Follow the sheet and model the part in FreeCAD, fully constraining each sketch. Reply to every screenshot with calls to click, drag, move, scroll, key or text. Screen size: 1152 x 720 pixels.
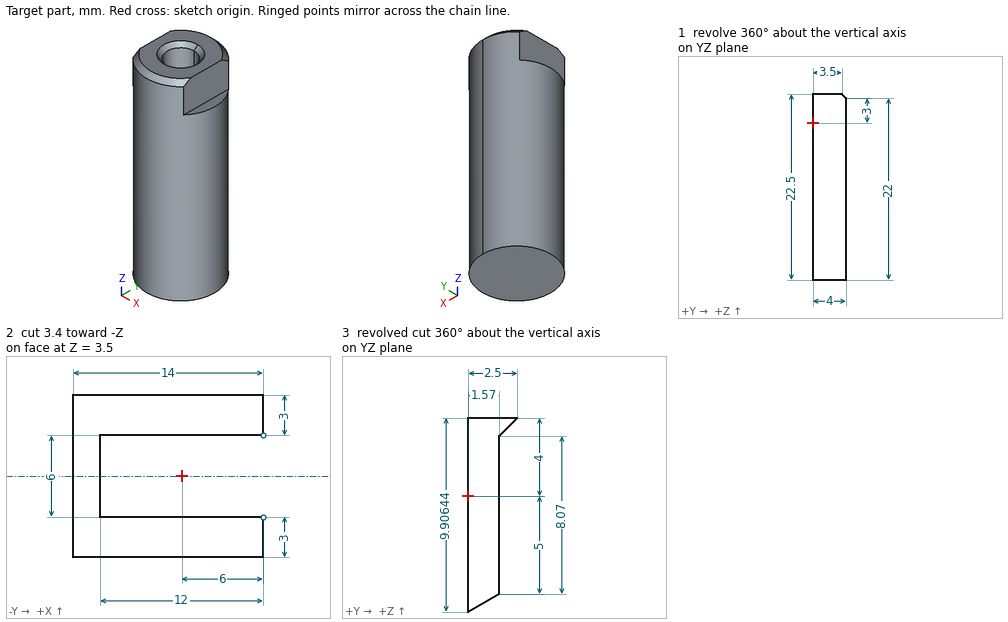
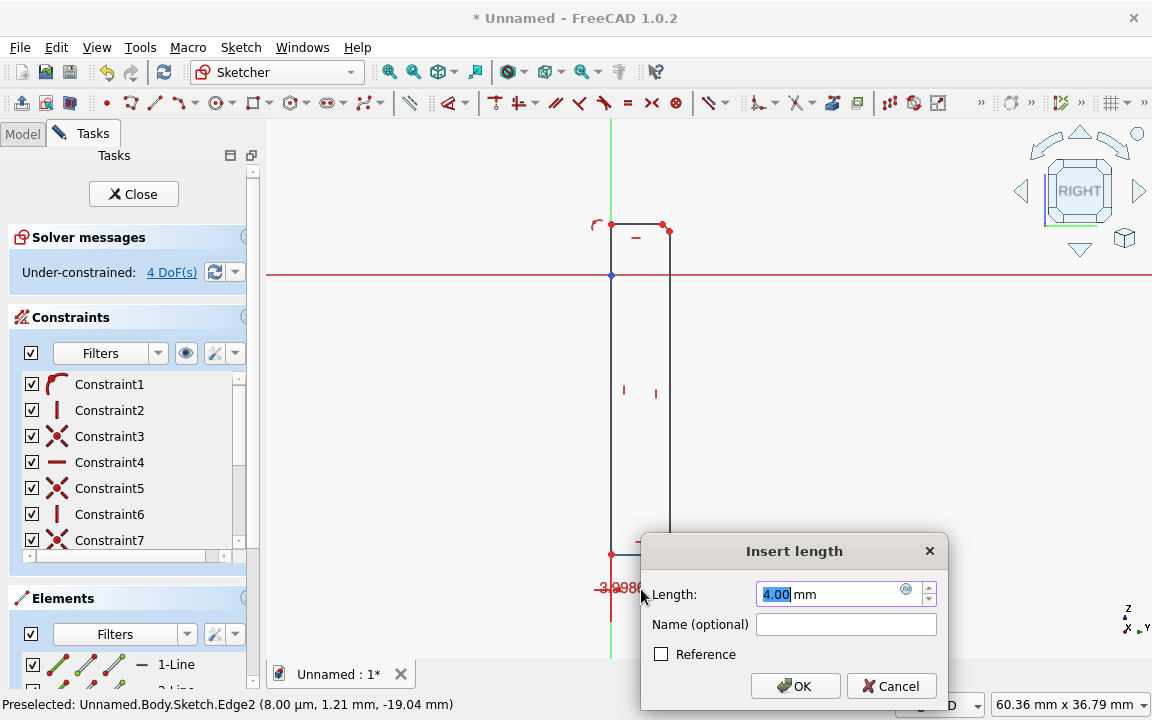
text(4)
key(Return)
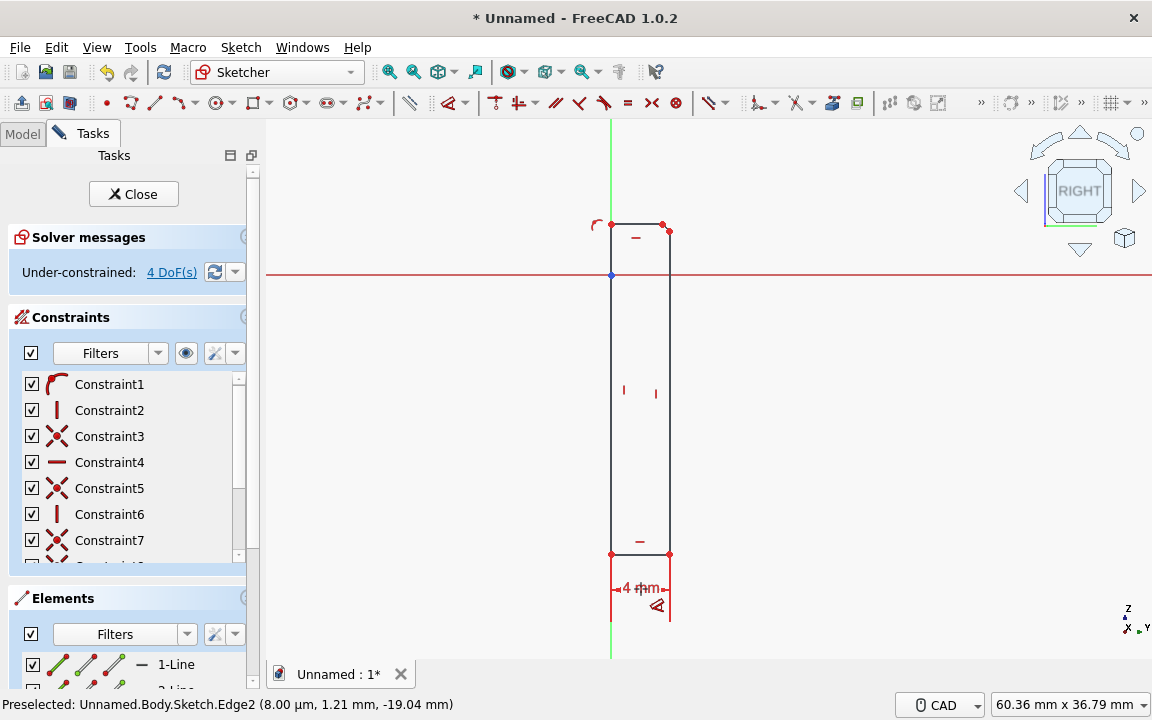
click(670, 458)
click(704, 393)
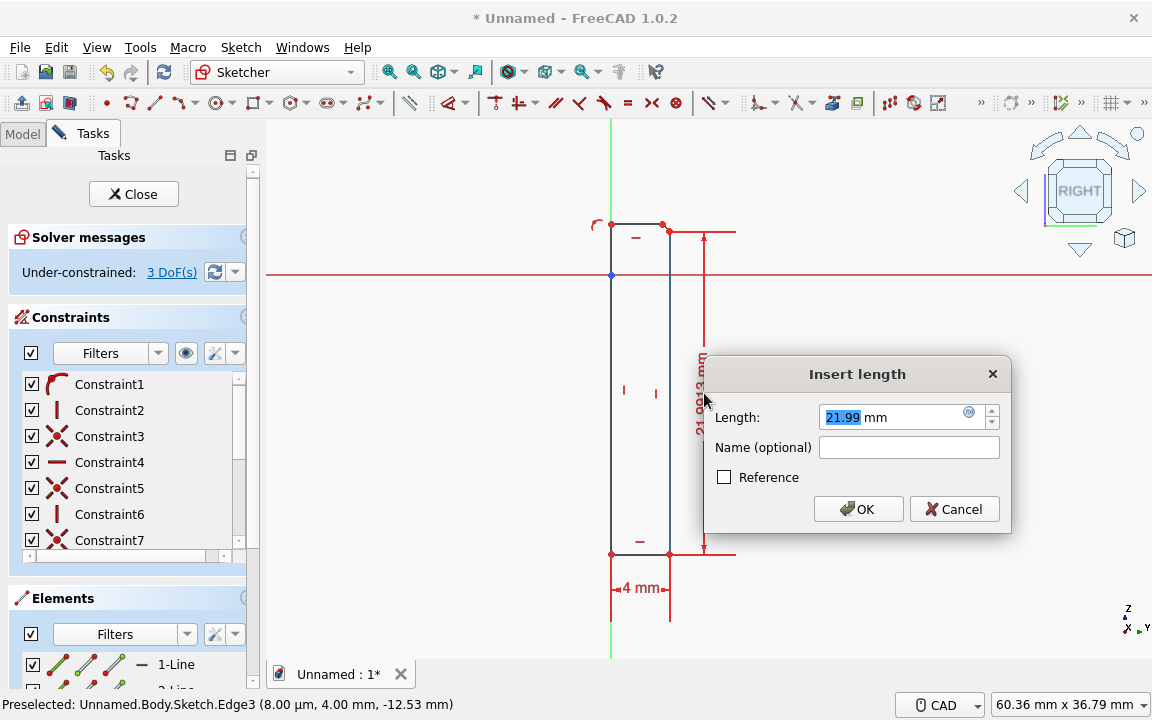
text(22)
key(Return)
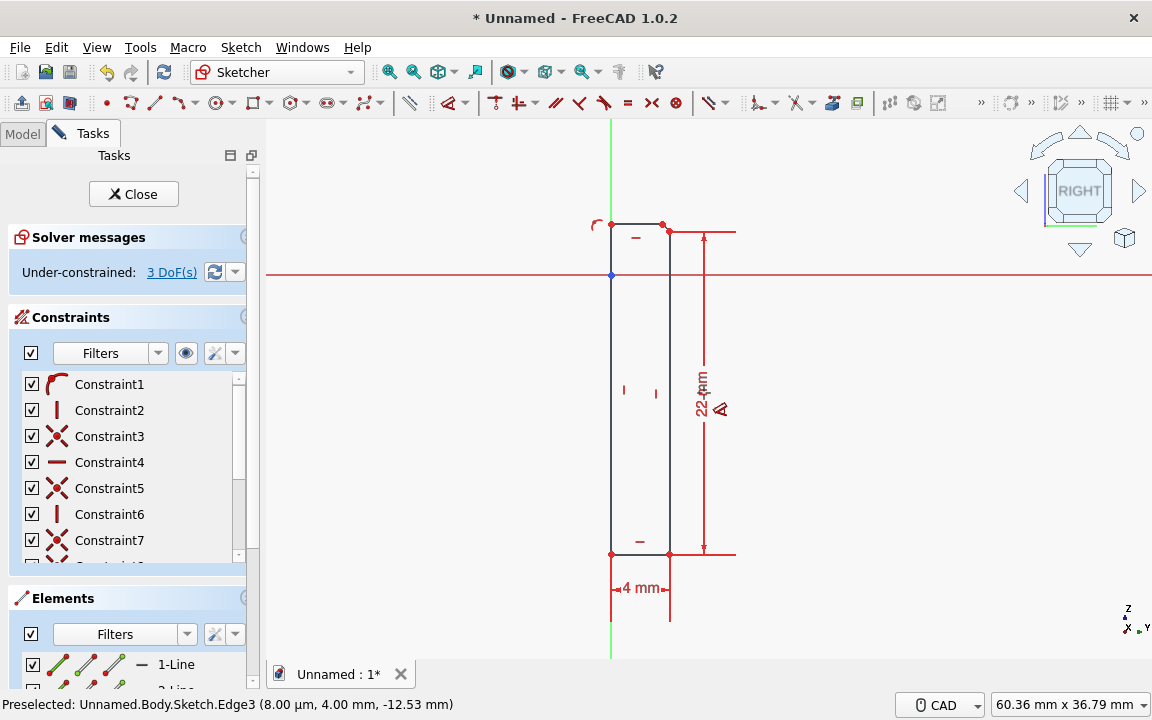
click(670, 232)
click(704, 253)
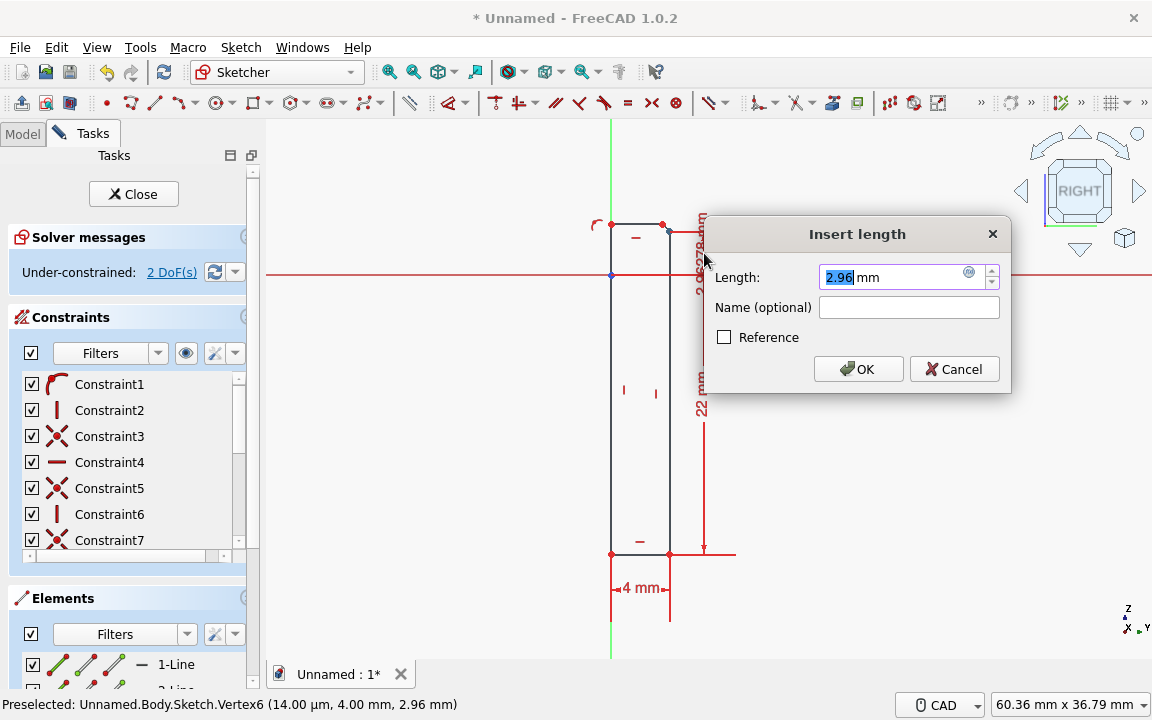
text(3)
key(Return)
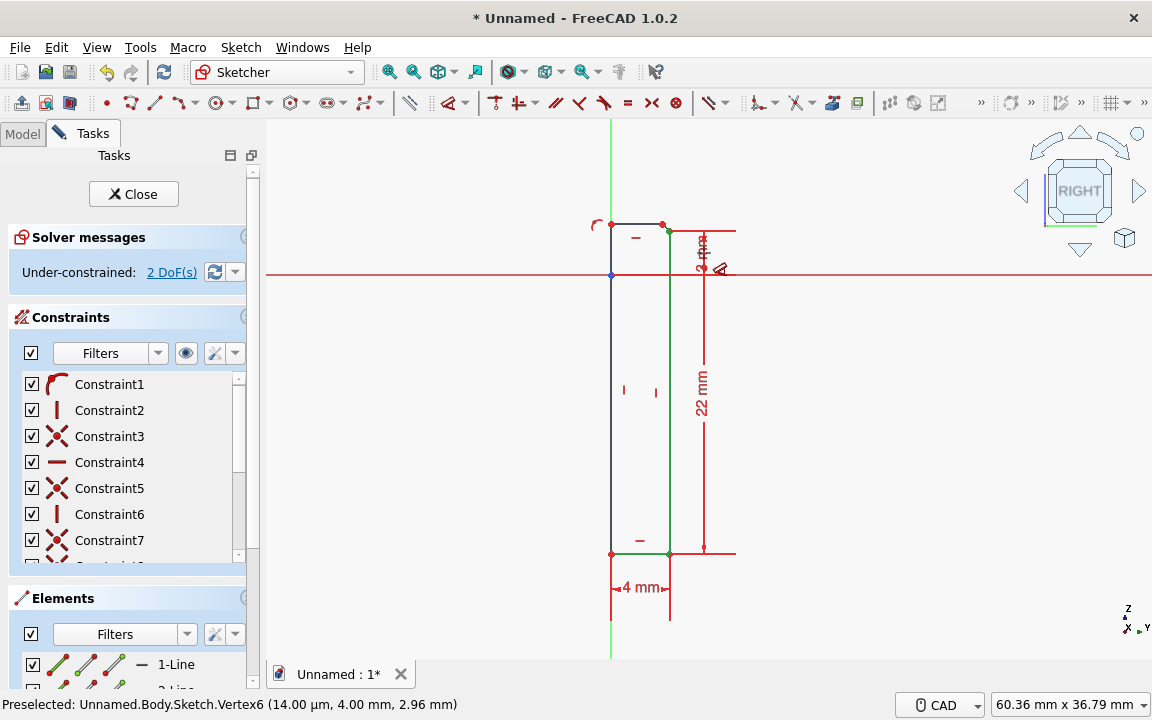
click(647, 224)
click(637, 190)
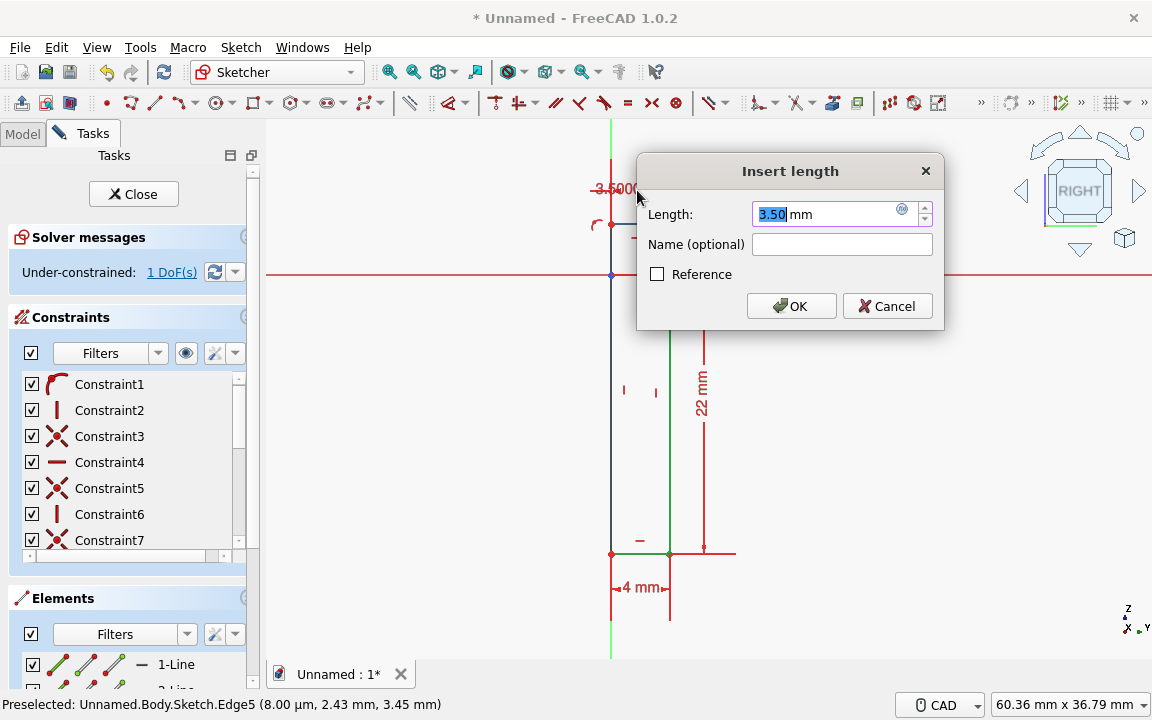
text(3.5)
key(Return)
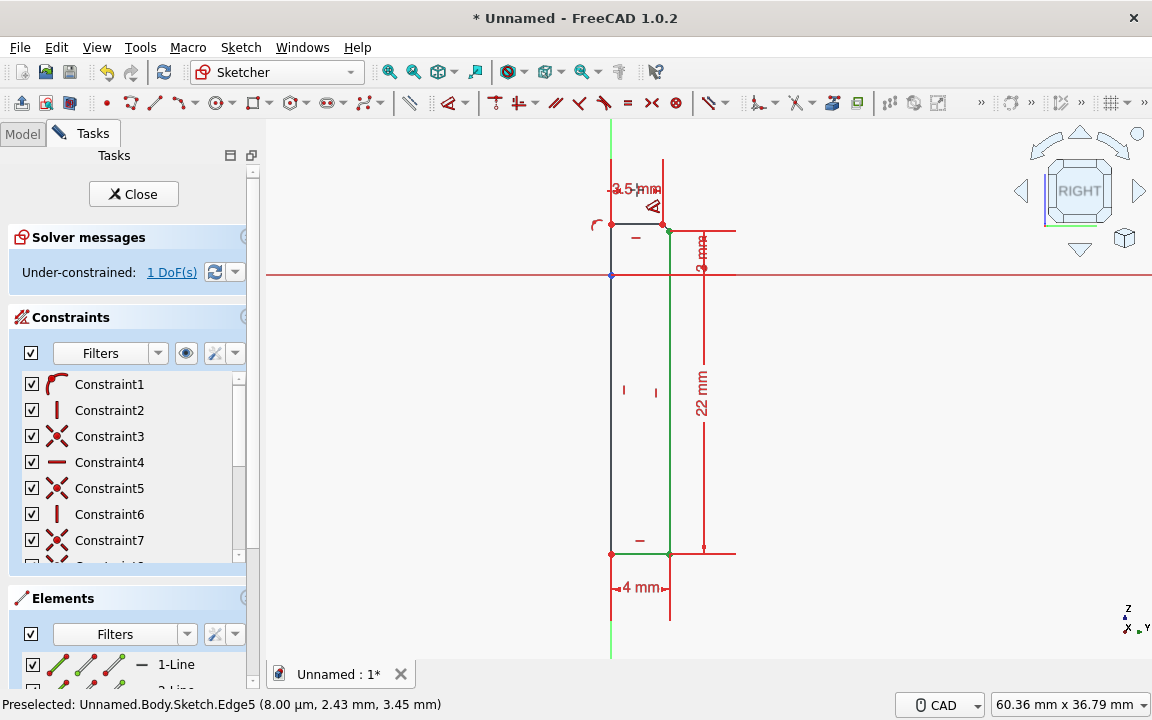
click(611, 323)
click(577, 389)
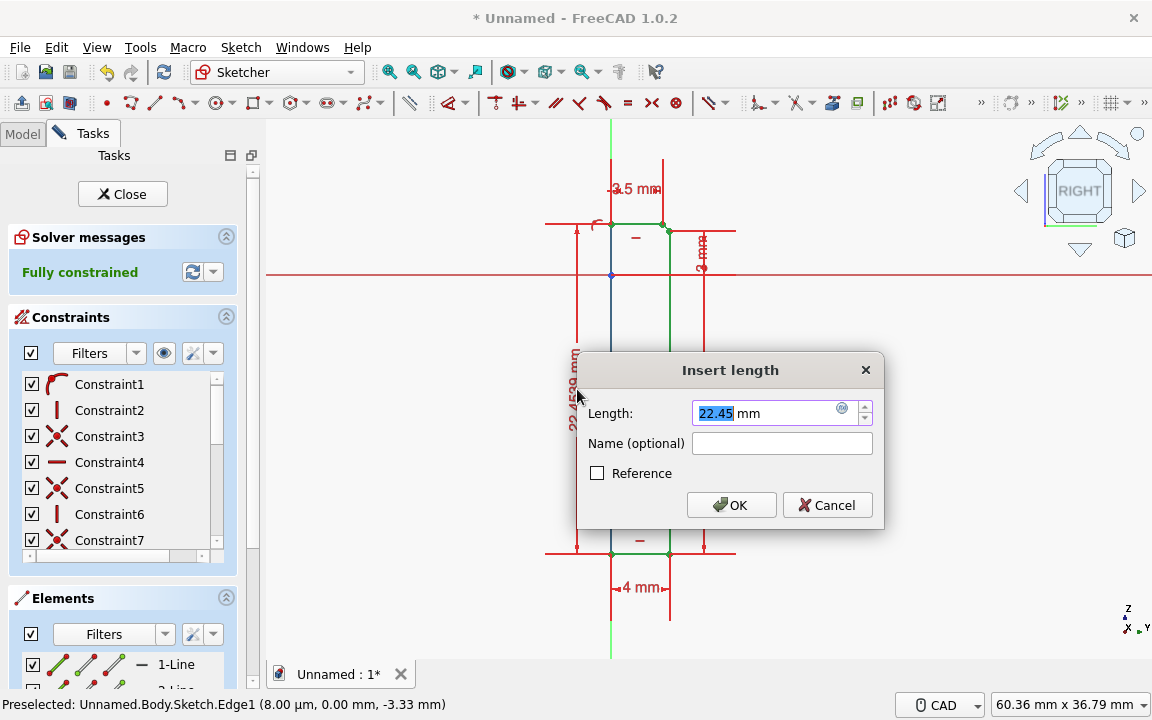
text(22.5)
key(Return)
key(Escape)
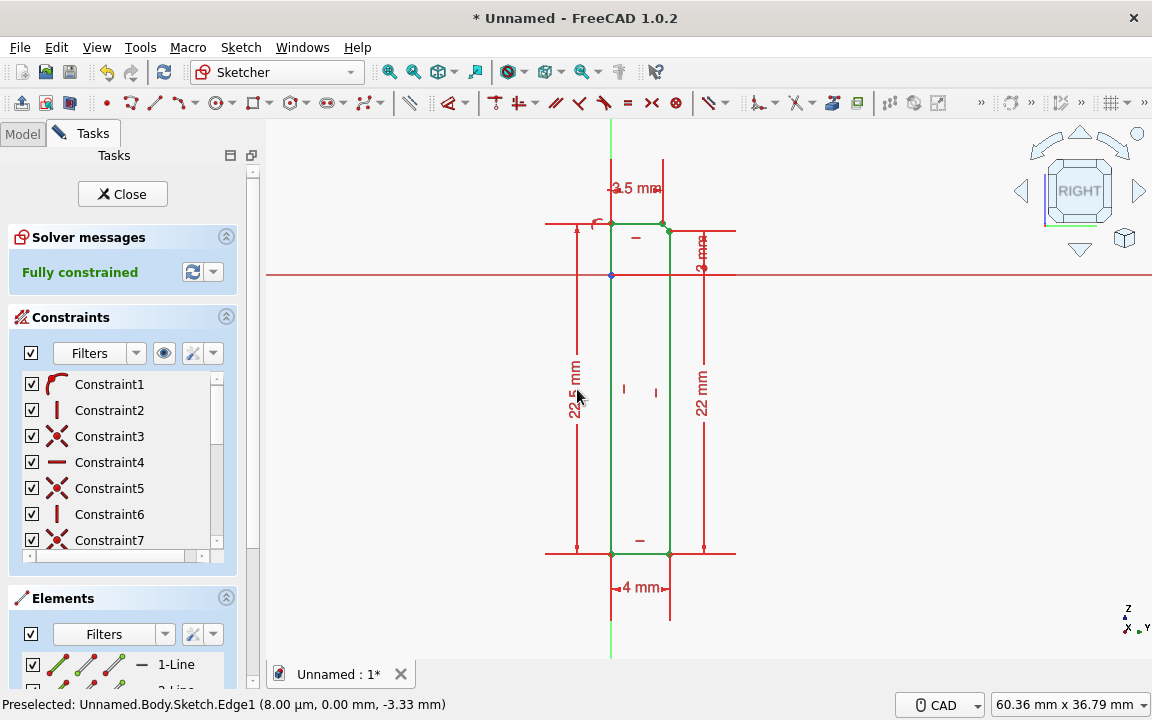
click(123, 194)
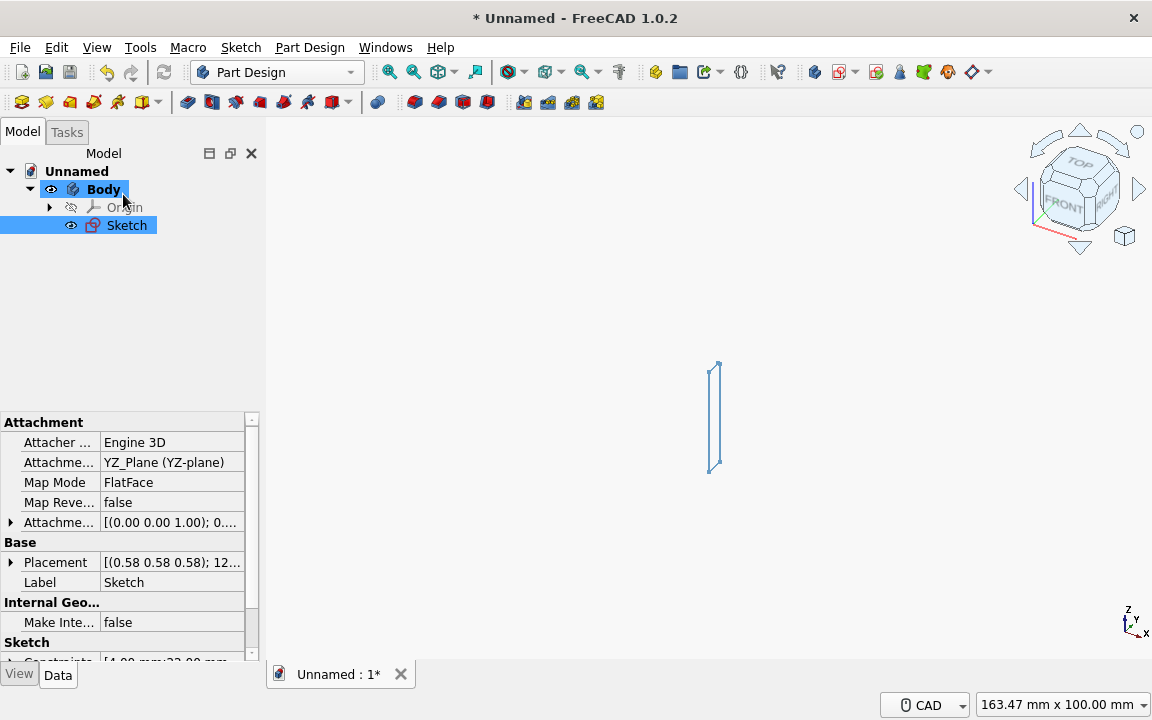
click(46, 102)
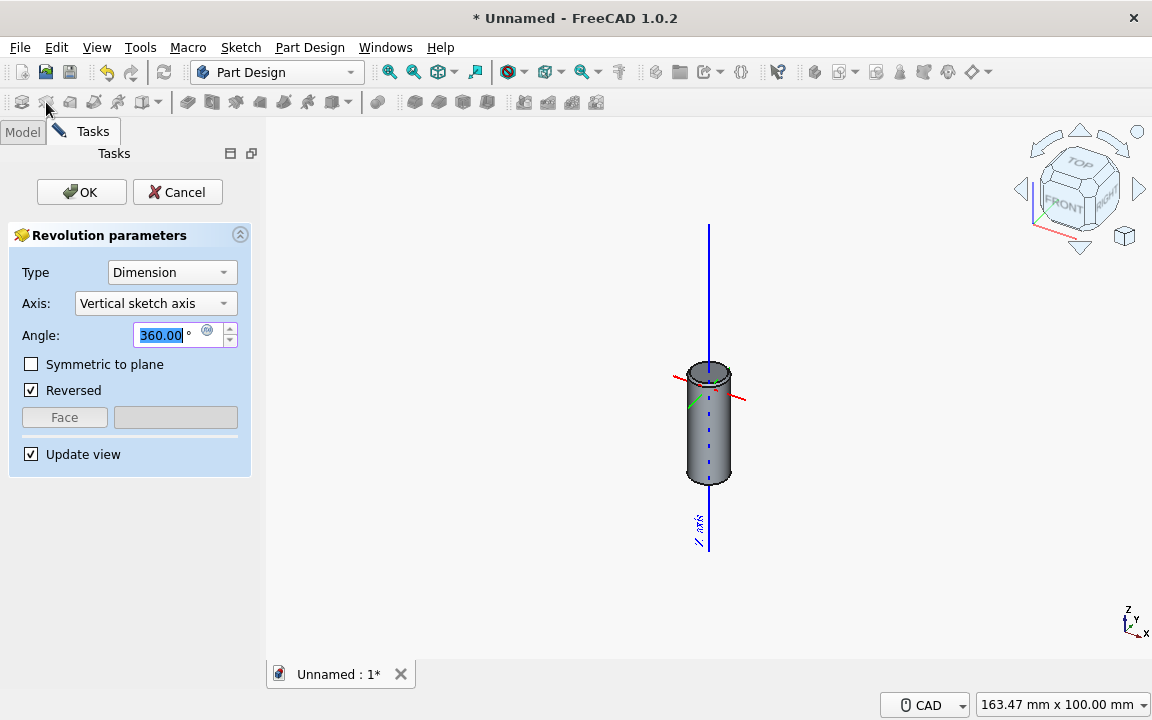
click(82, 192)